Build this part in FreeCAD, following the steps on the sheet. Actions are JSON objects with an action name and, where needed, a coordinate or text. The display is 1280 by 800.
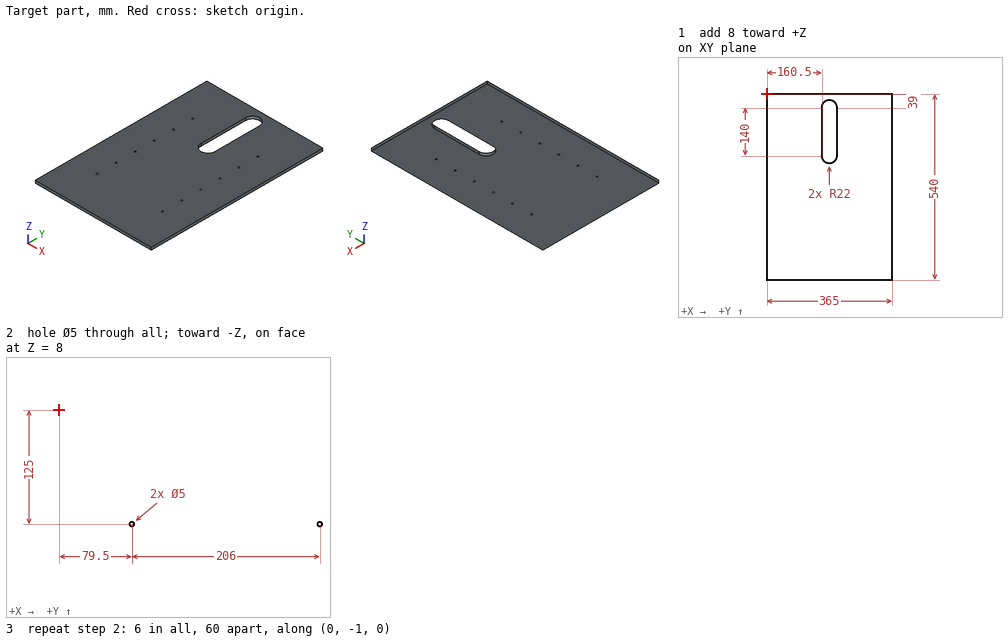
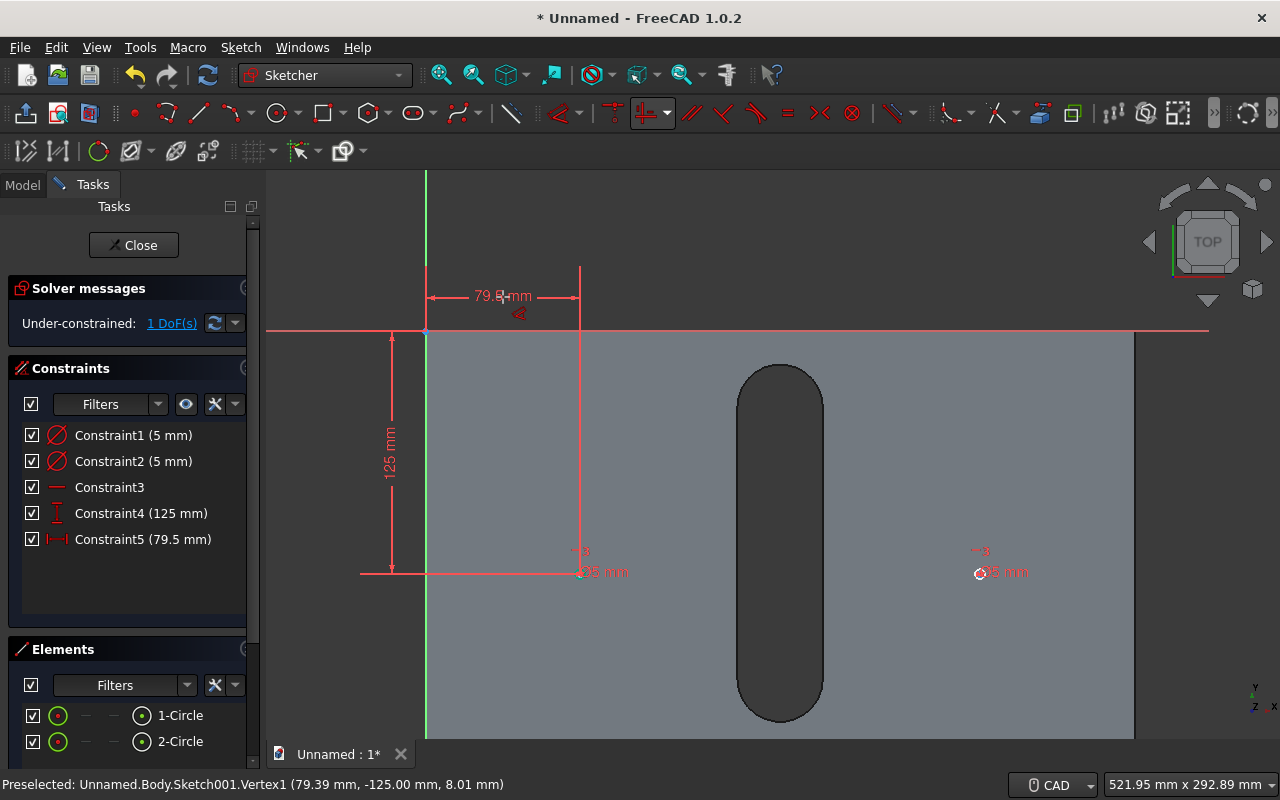
{"action": "left_click", "coordinate": [580, 574]}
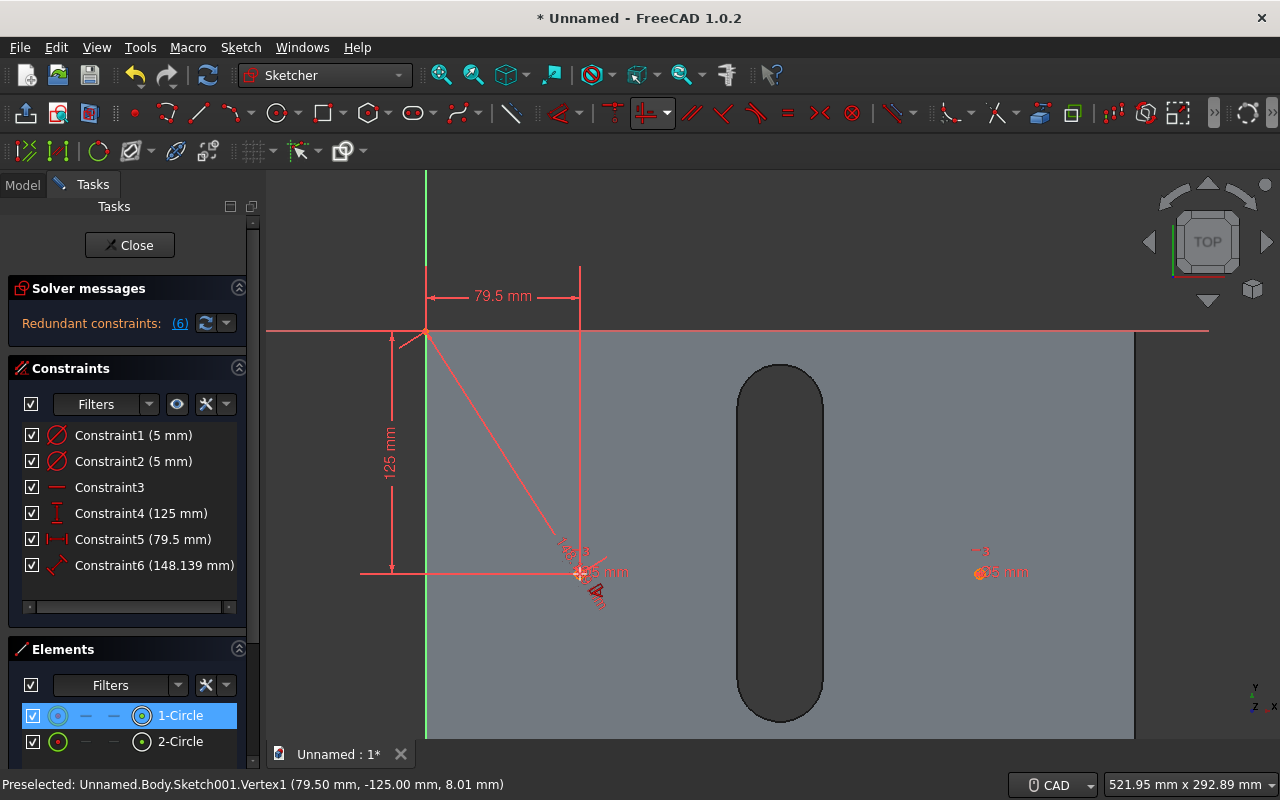
{"action": "left_click", "coordinate": [980, 574]}
{"action": "left_click", "coordinate": [780, 608]}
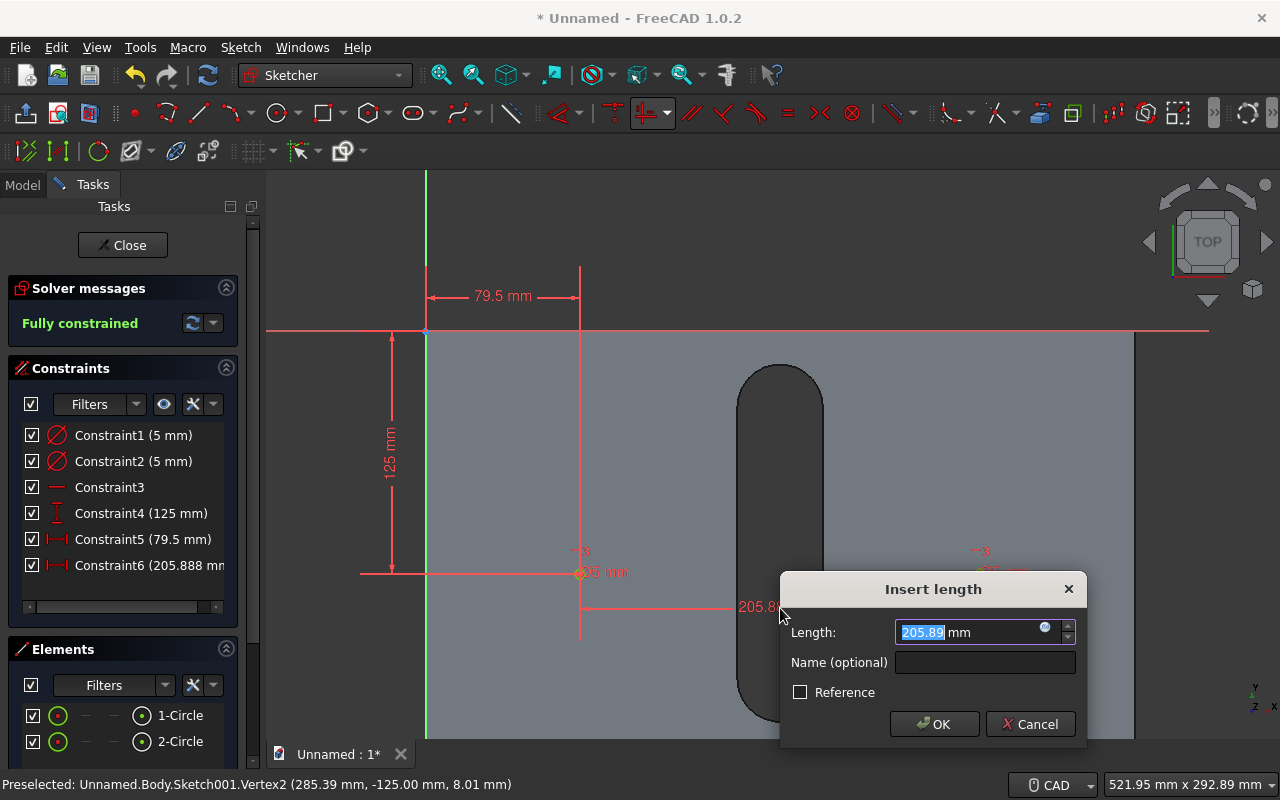
{"action": "type", "text": "206"}
{"action": "key", "text": "Return"}
{"action": "key", "text": "Escape"}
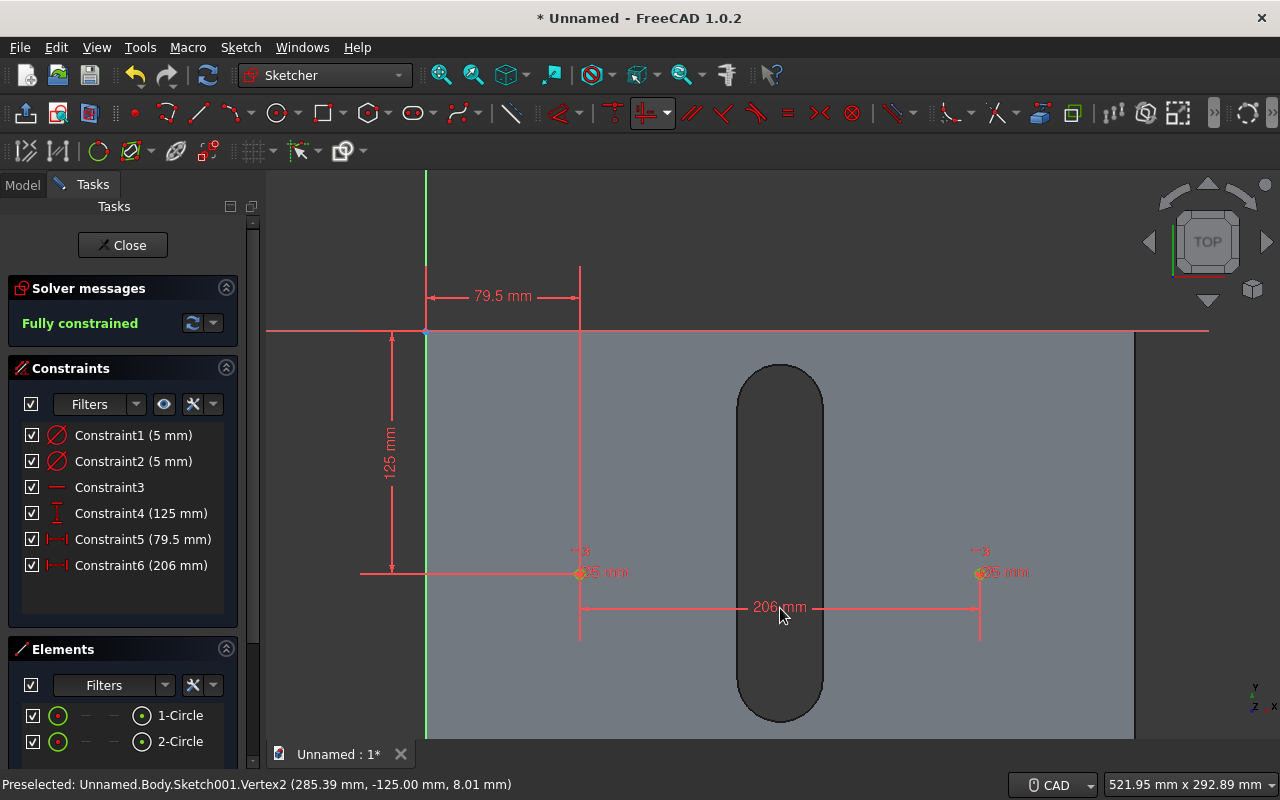
{"action": "left_click", "coordinate": [123, 245]}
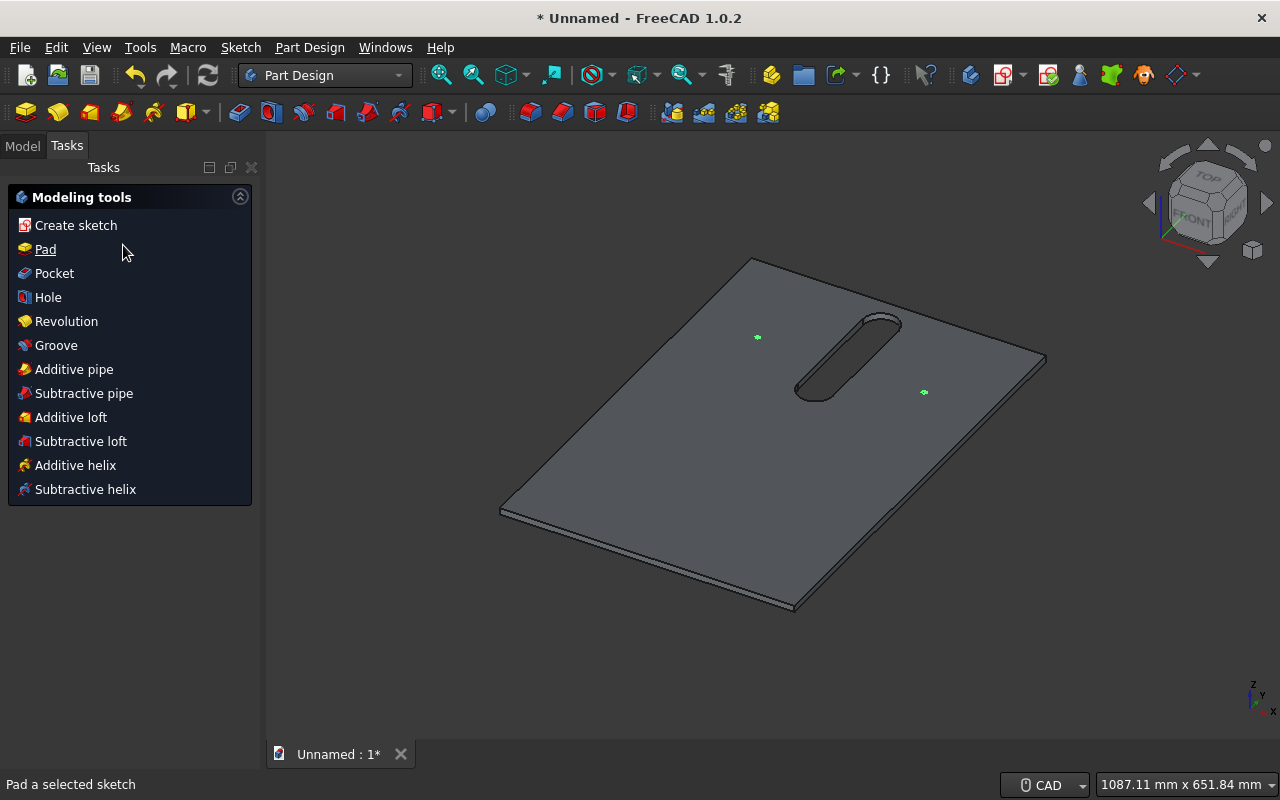
{"action": "left_click", "coordinate": [272, 112]}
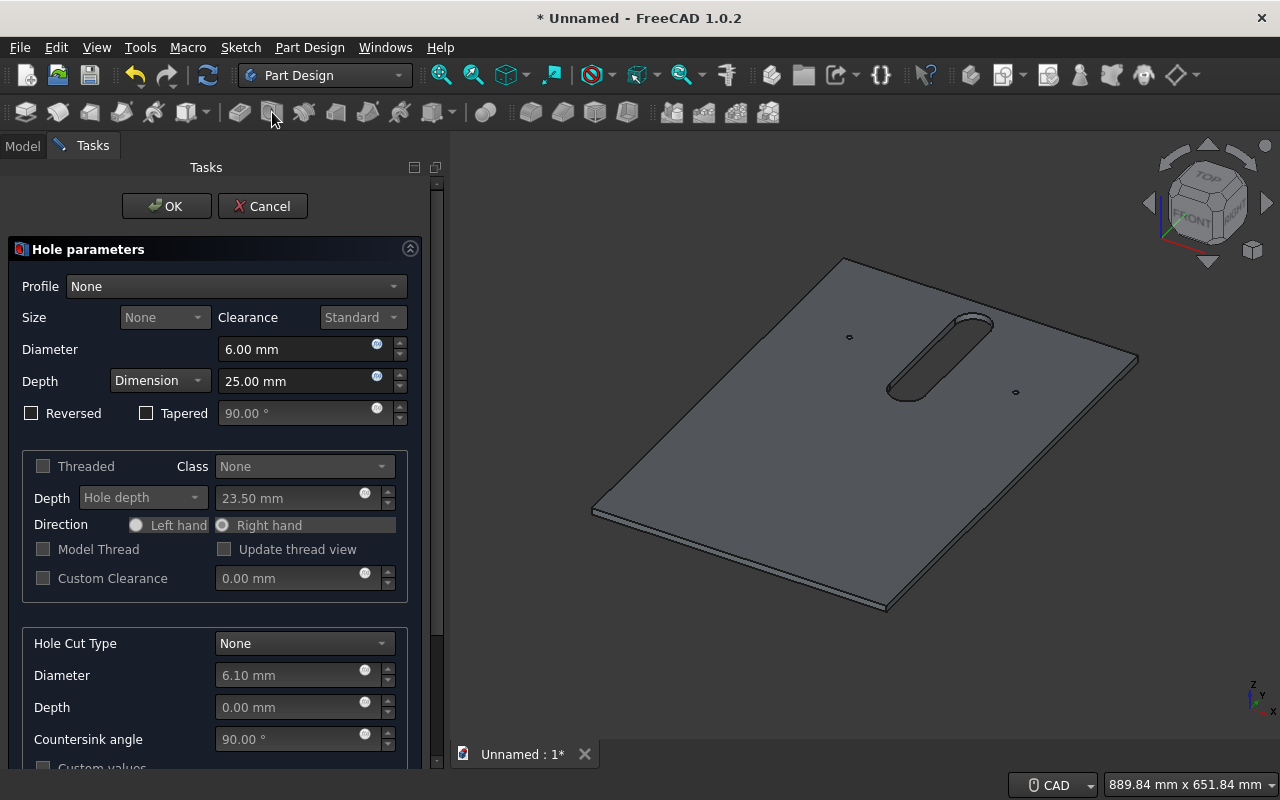
{"action": "triple_click", "coordinate": [305, 349]}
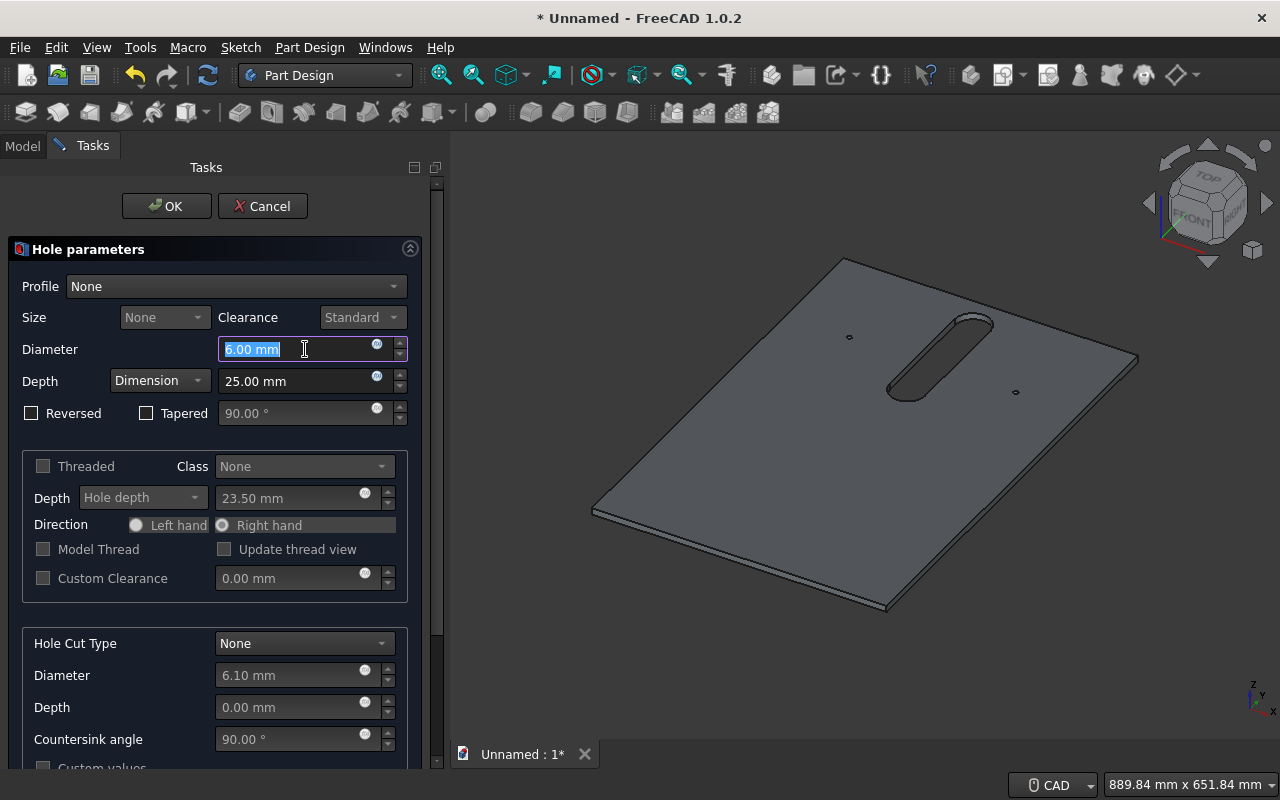
{"action": "type", "text": "5"}
{"action": "key", "text": "Tab"}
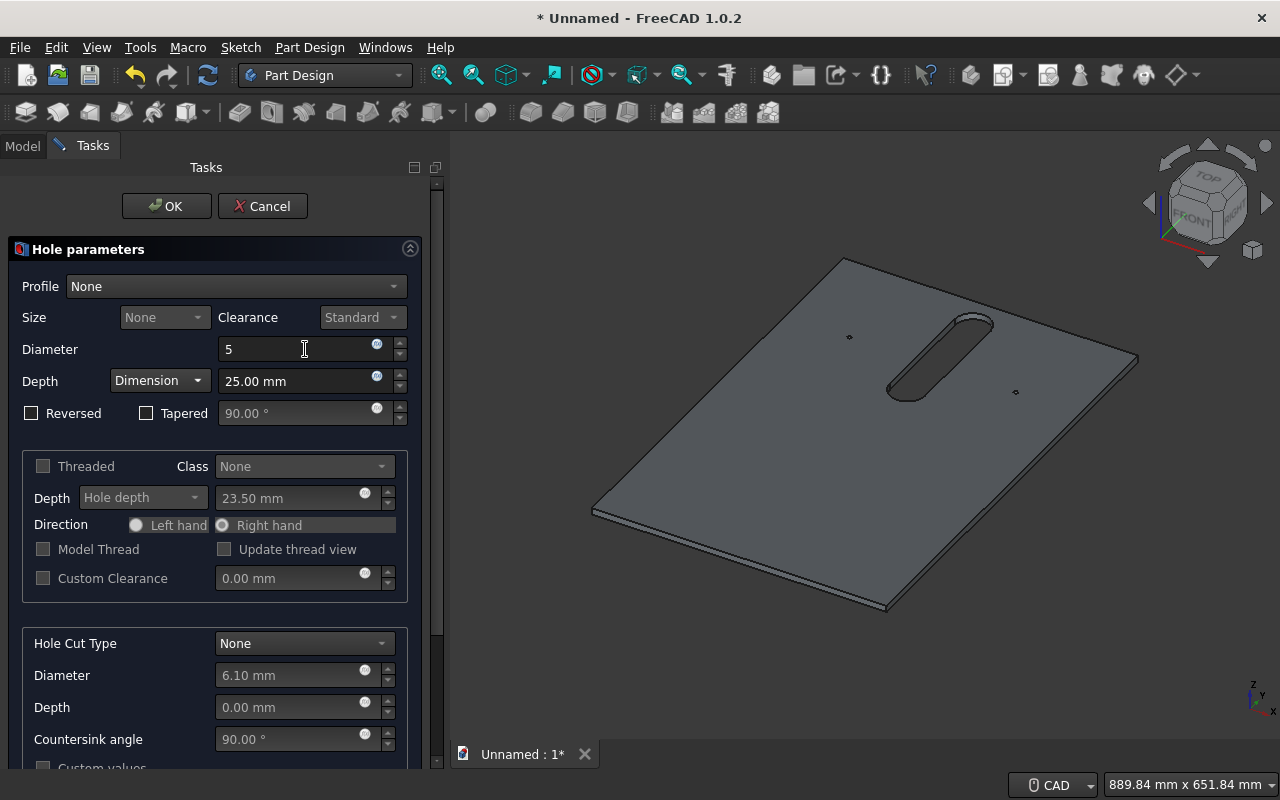
{"action": "left_click", "coordinate": [161, 380]}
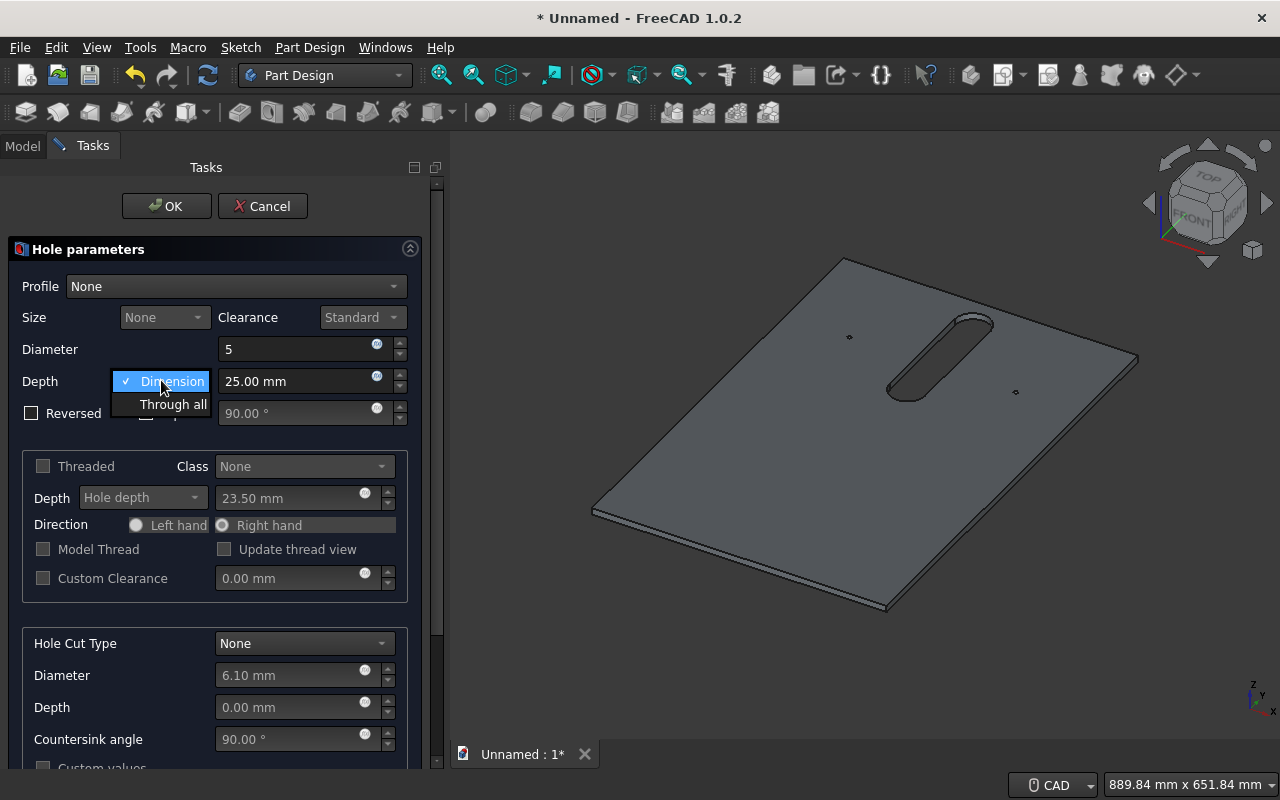
{"action": "left_click", "coordinate": [160, 404]}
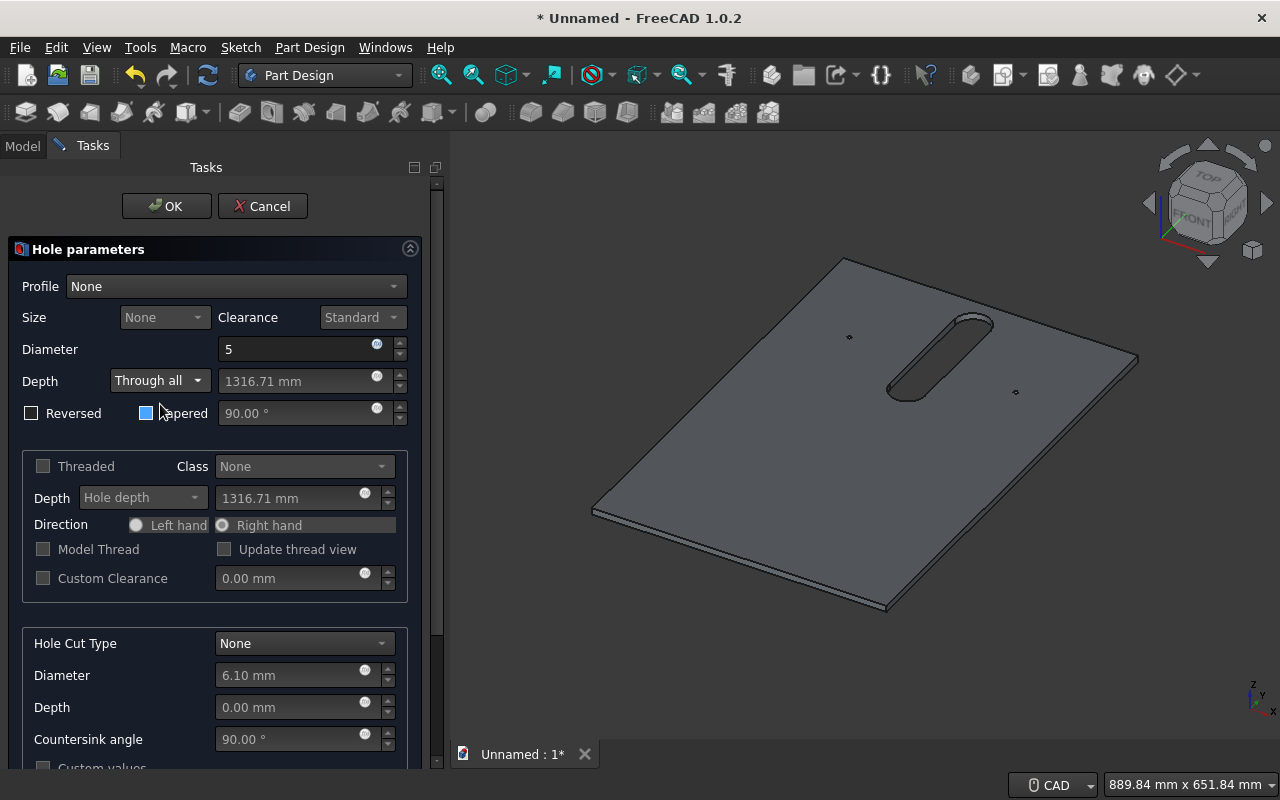
{"action": "left_click", "coordinate": [167, 206]}